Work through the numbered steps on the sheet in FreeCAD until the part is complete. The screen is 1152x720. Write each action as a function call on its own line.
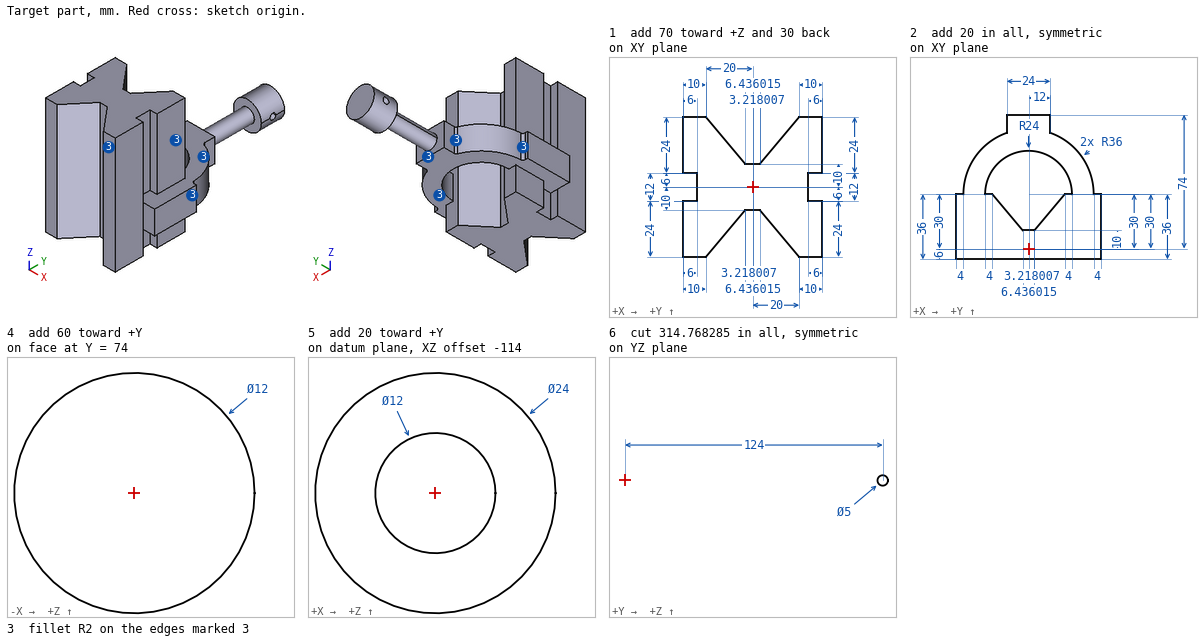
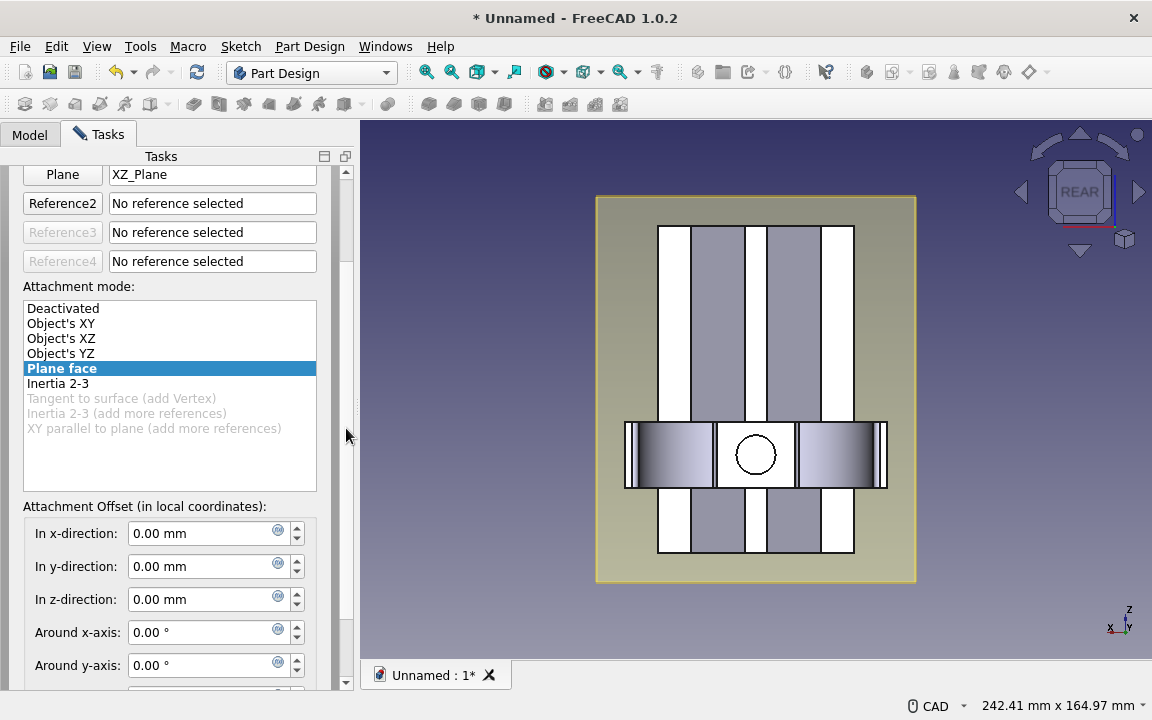
triple_click(210, 600)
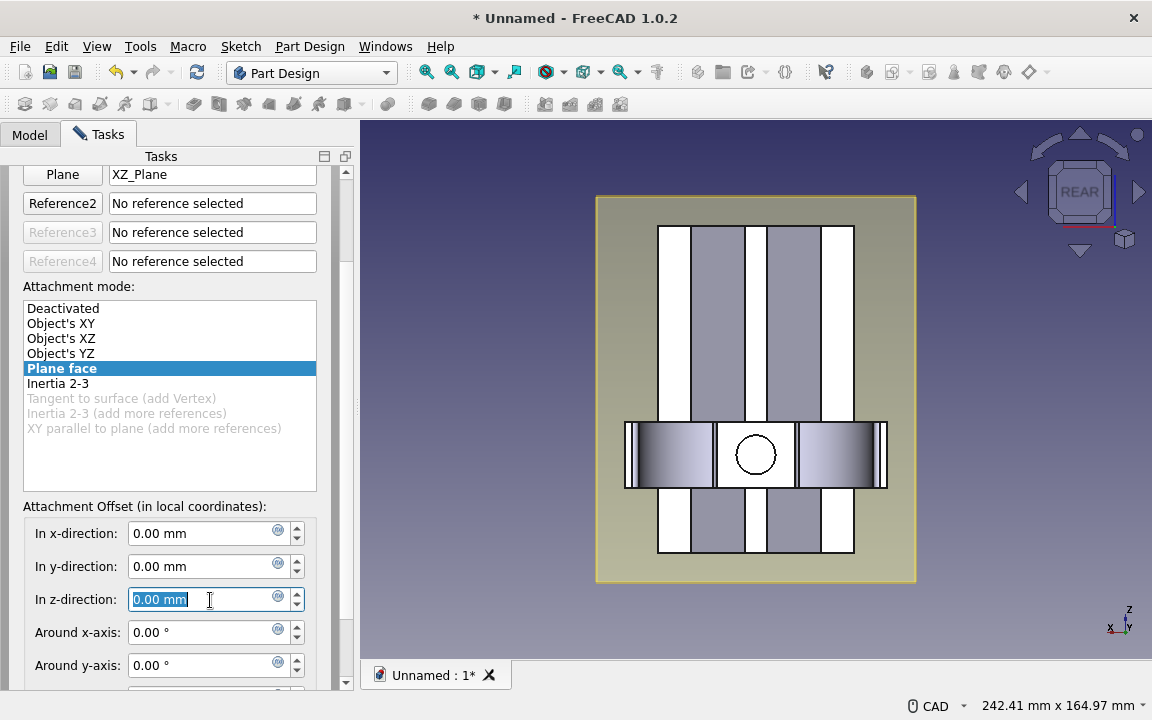
text(-114)
key(Tab)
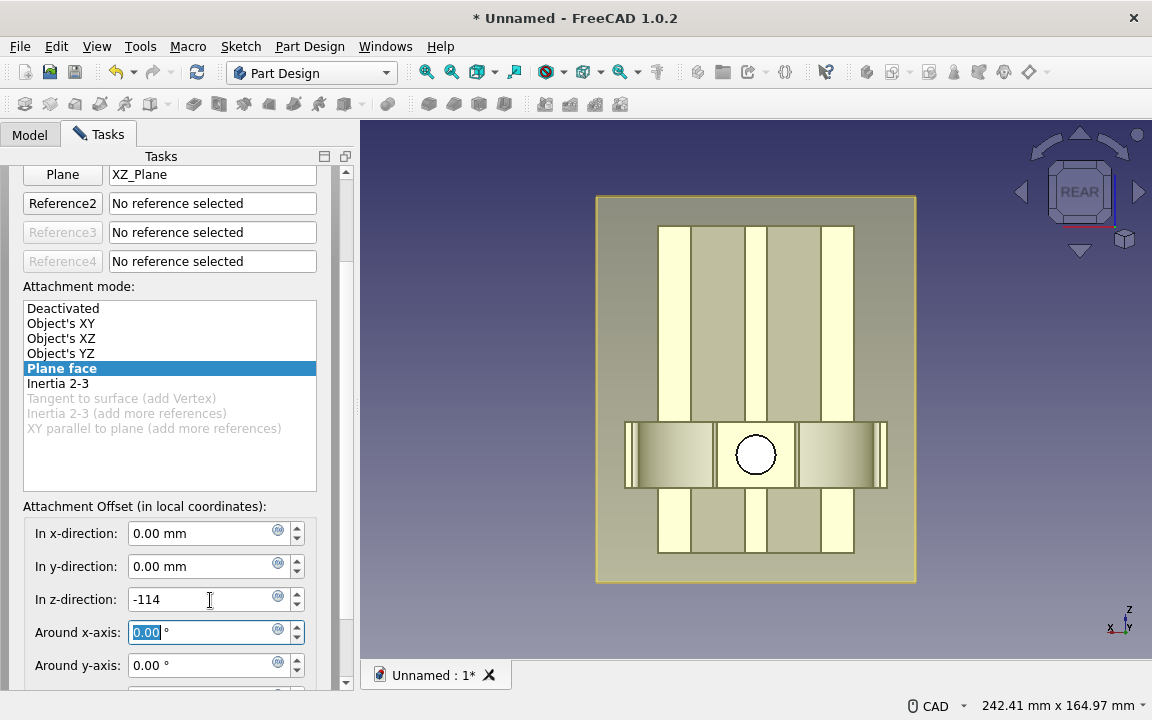
scroll(346, 428, up, 3)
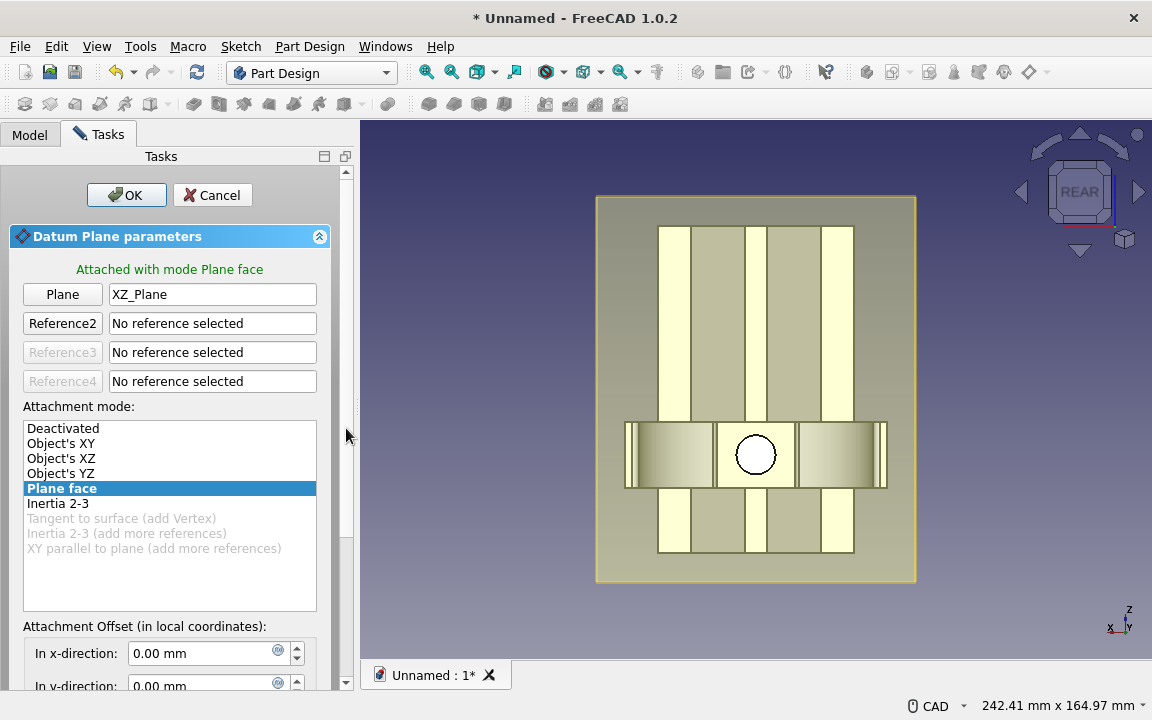
click(127, 195)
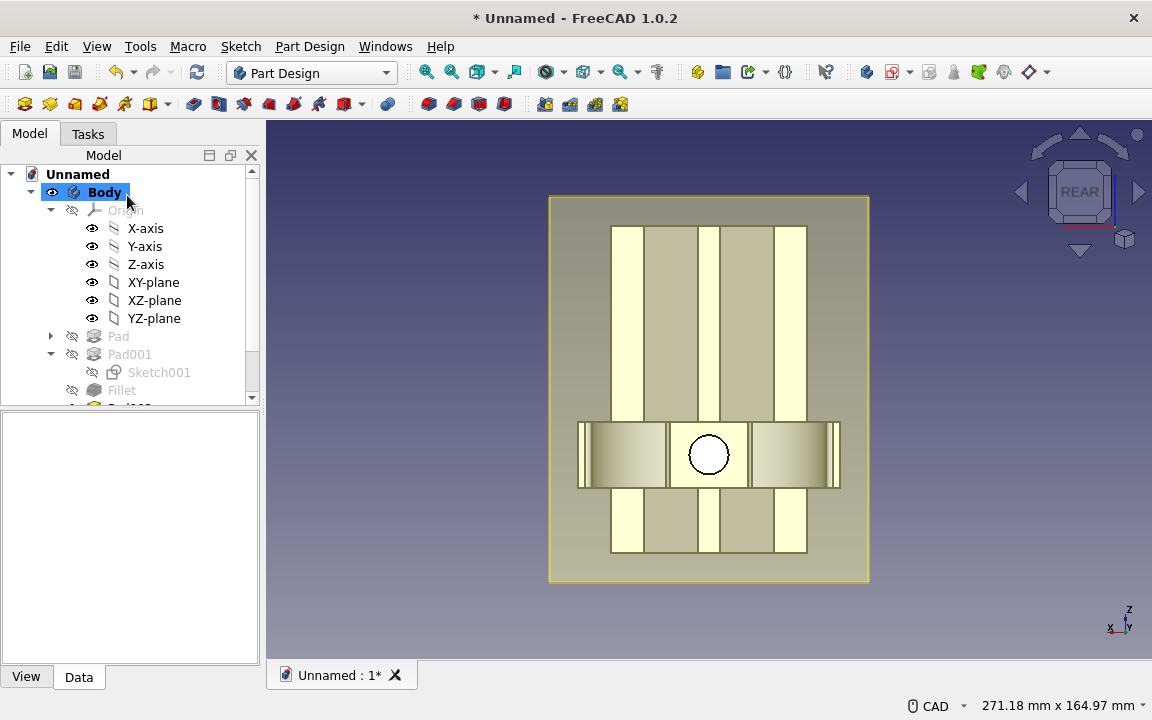
scroll(101, 278, down, 3)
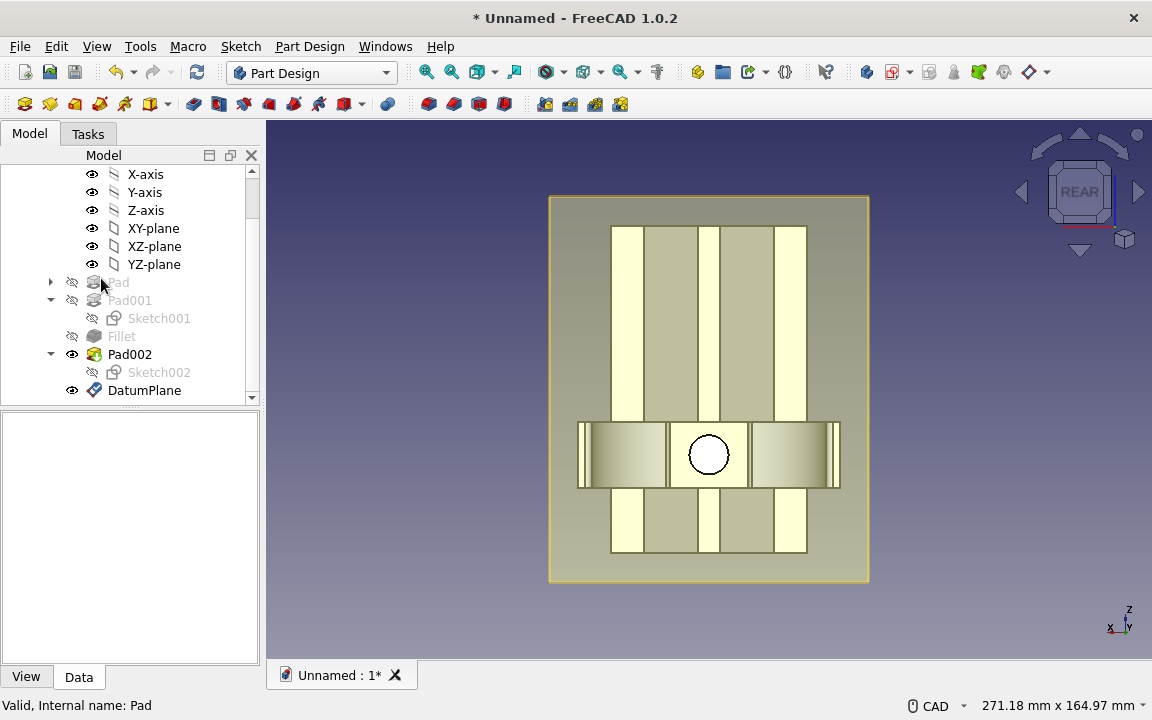
click(117, 390)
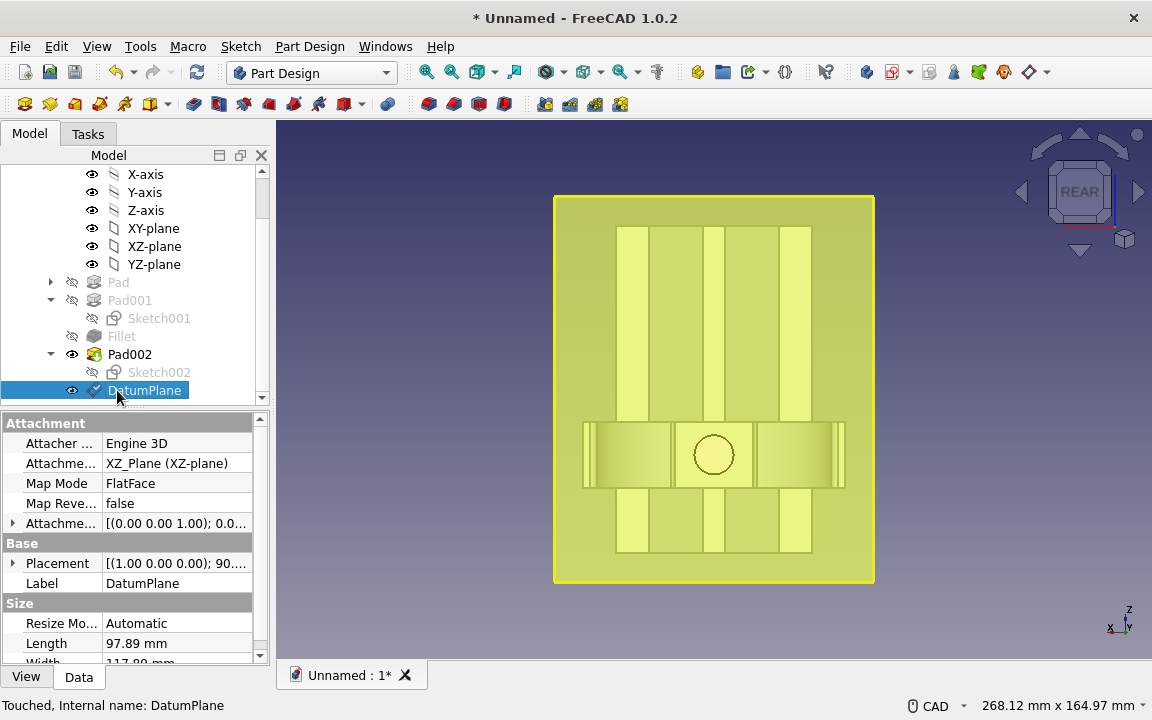
click(892, 72)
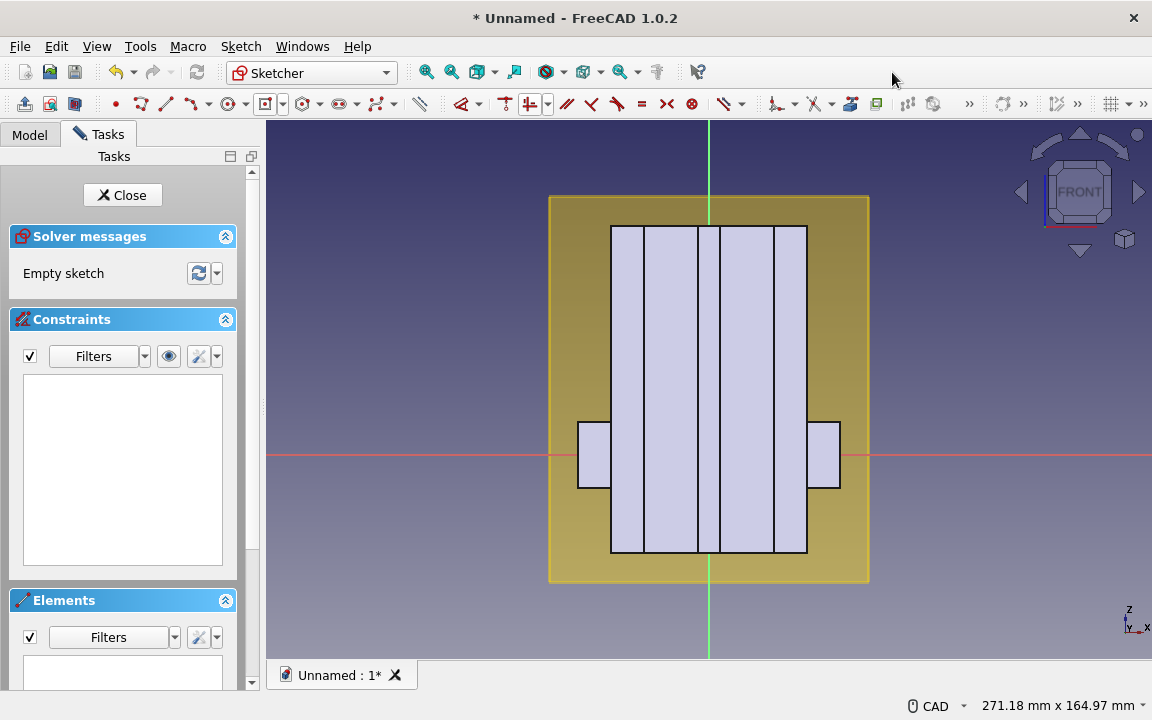
click(75, 104)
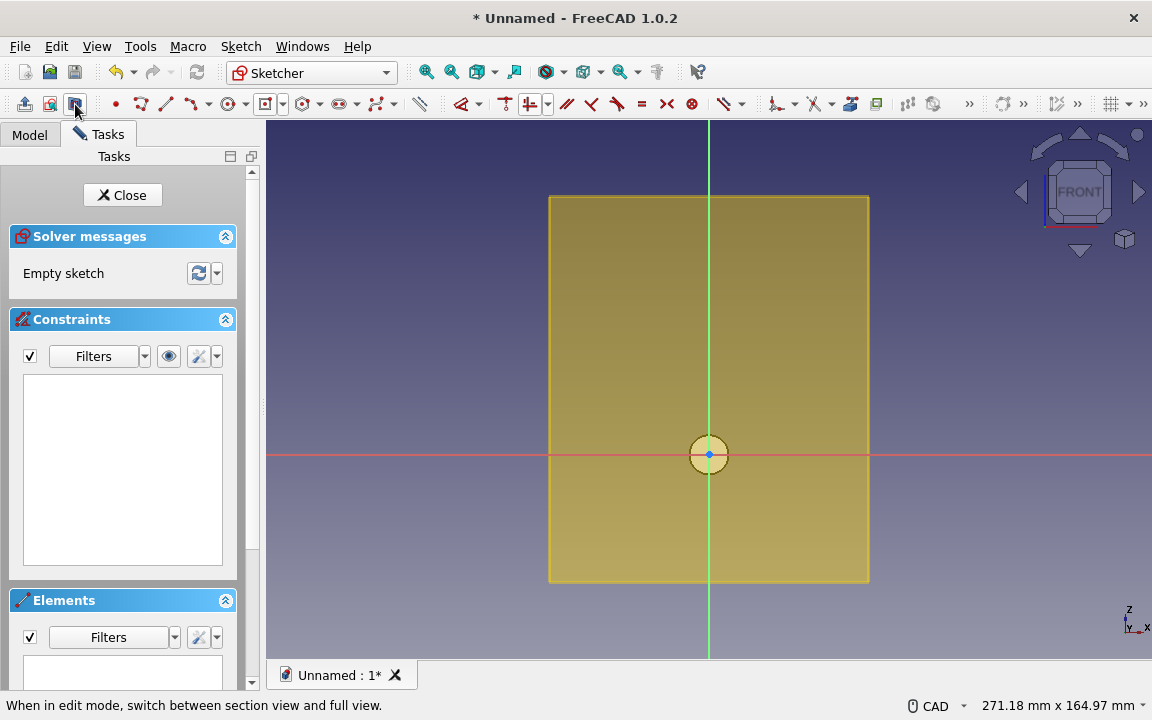
scroll(731, 476, up, 7)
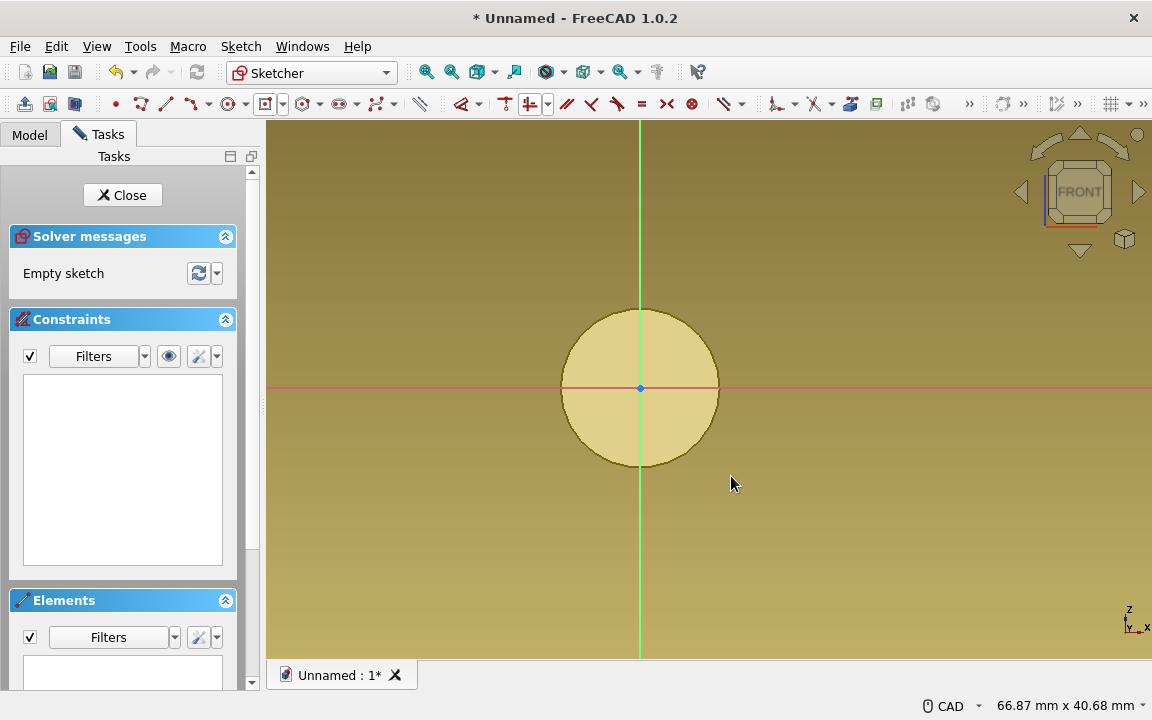
click(228, 104)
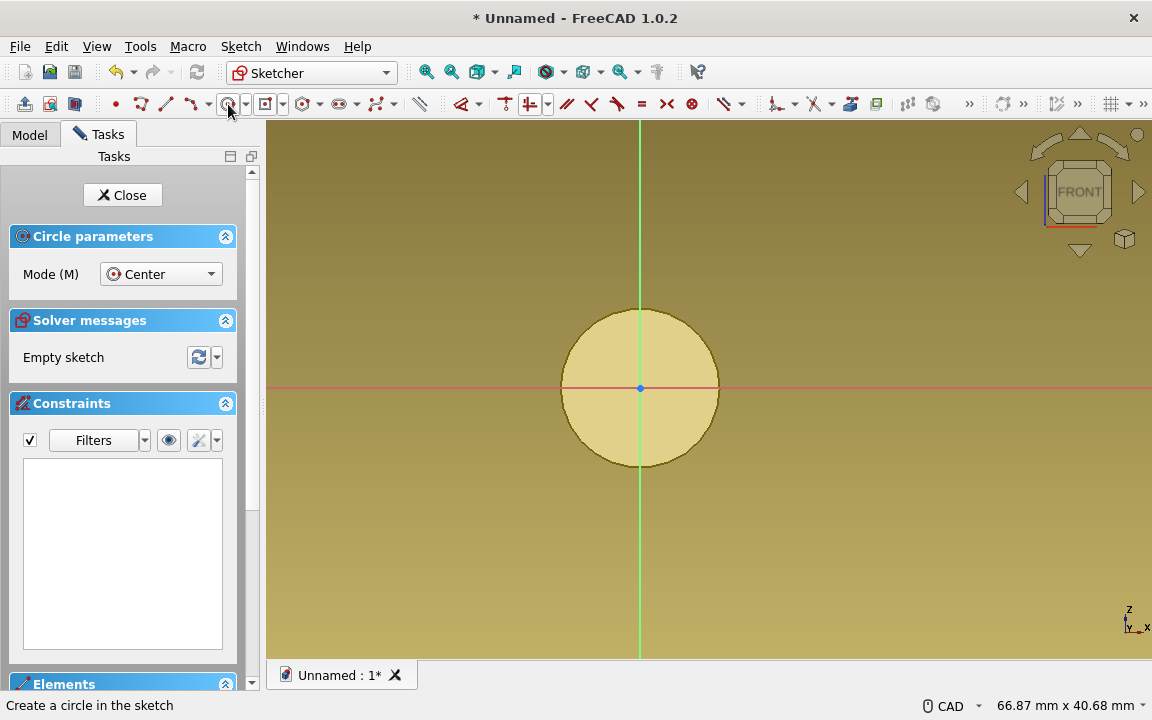
click(640, 388)
move(753, 276)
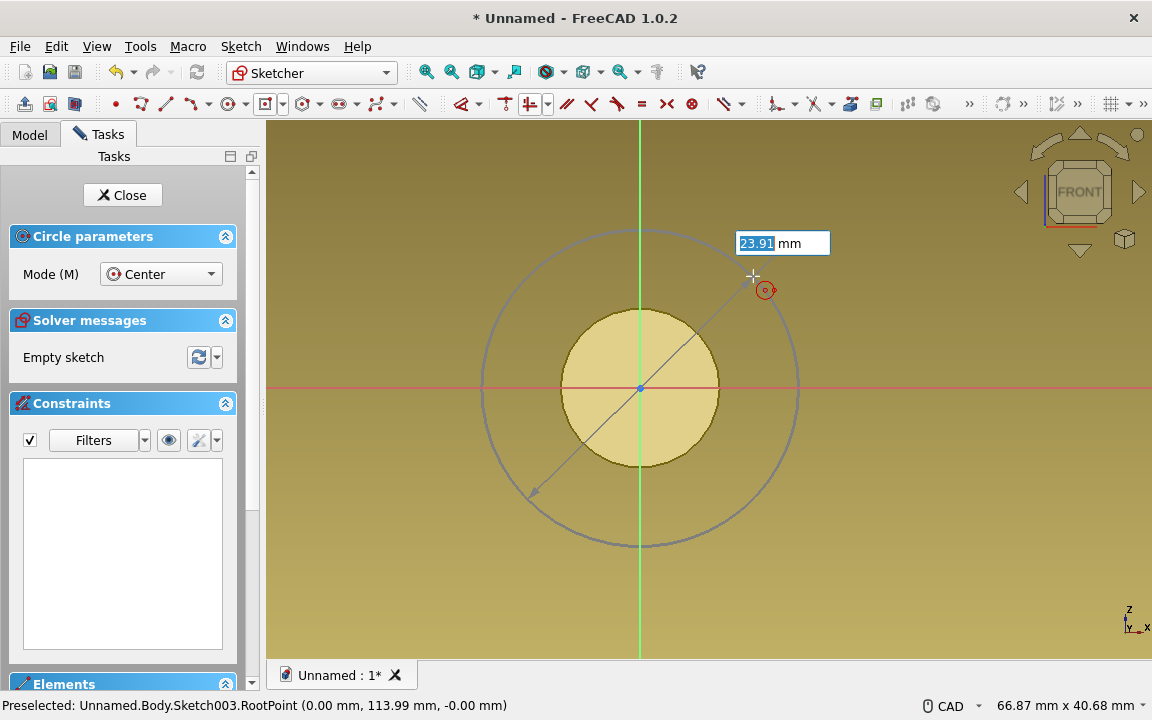
text(24)
key(Return)